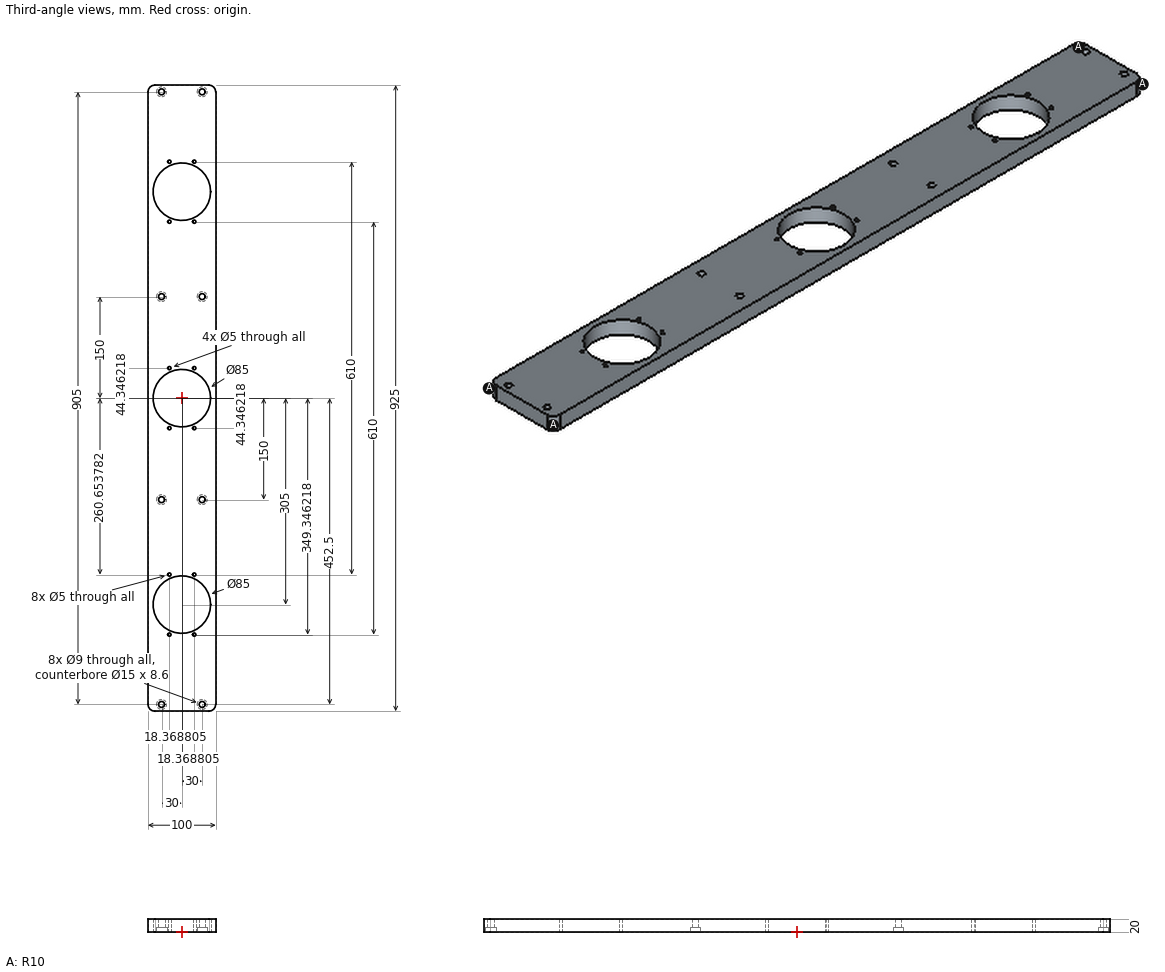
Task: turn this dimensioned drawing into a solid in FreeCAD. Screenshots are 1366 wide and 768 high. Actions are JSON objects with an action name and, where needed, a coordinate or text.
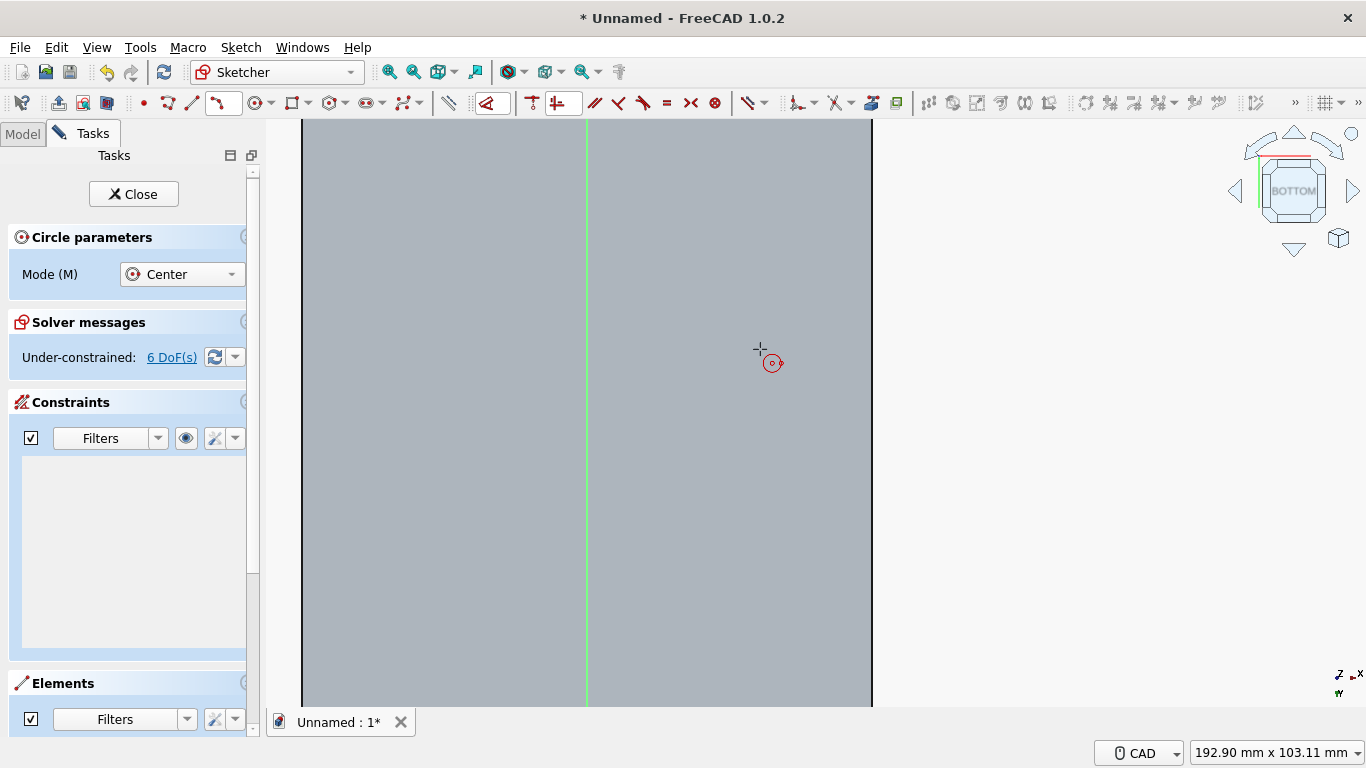
{"action": "scroll", "coordinate": [760, 349], "scroll_direction": "down", "scroll_amount": 13}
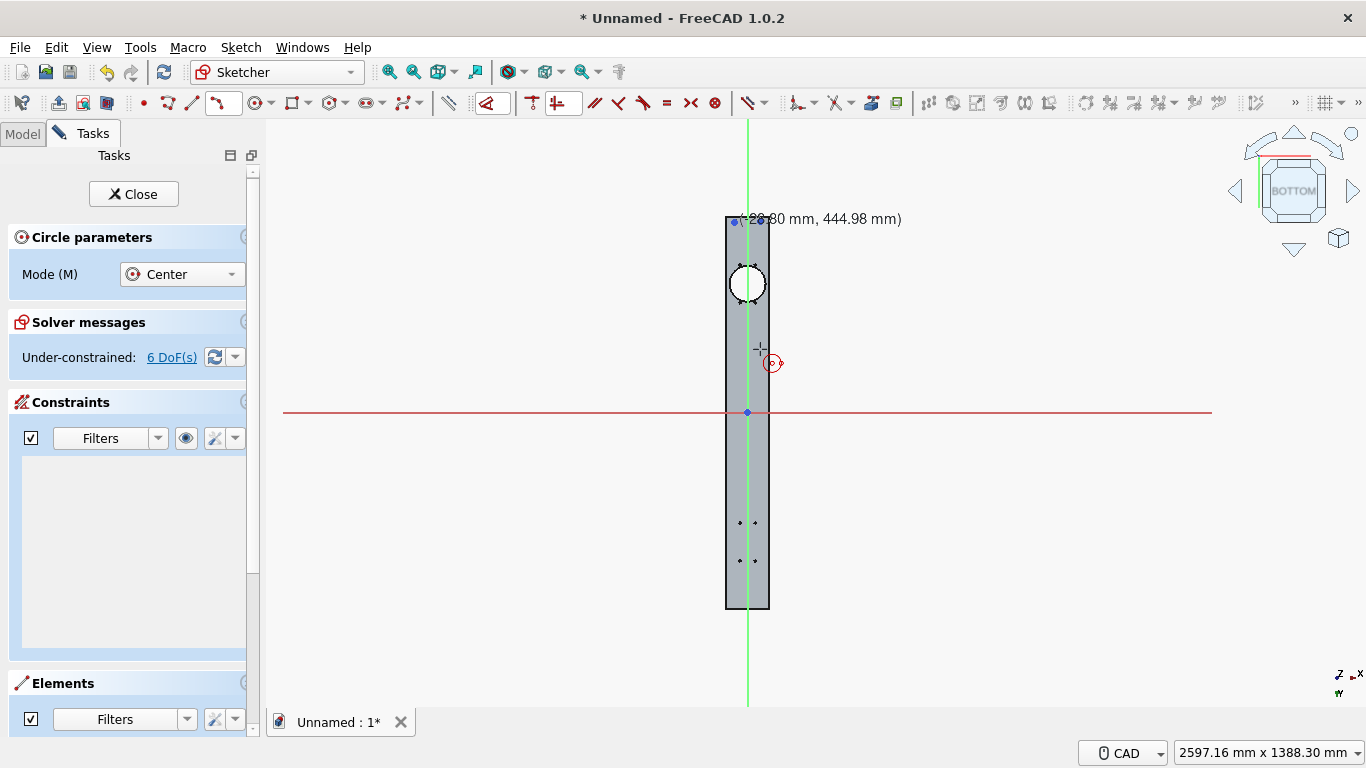
{"action": "scroll", "coordinate": [760, 349], "scroll_direction": "up", "scroll_amount": 2}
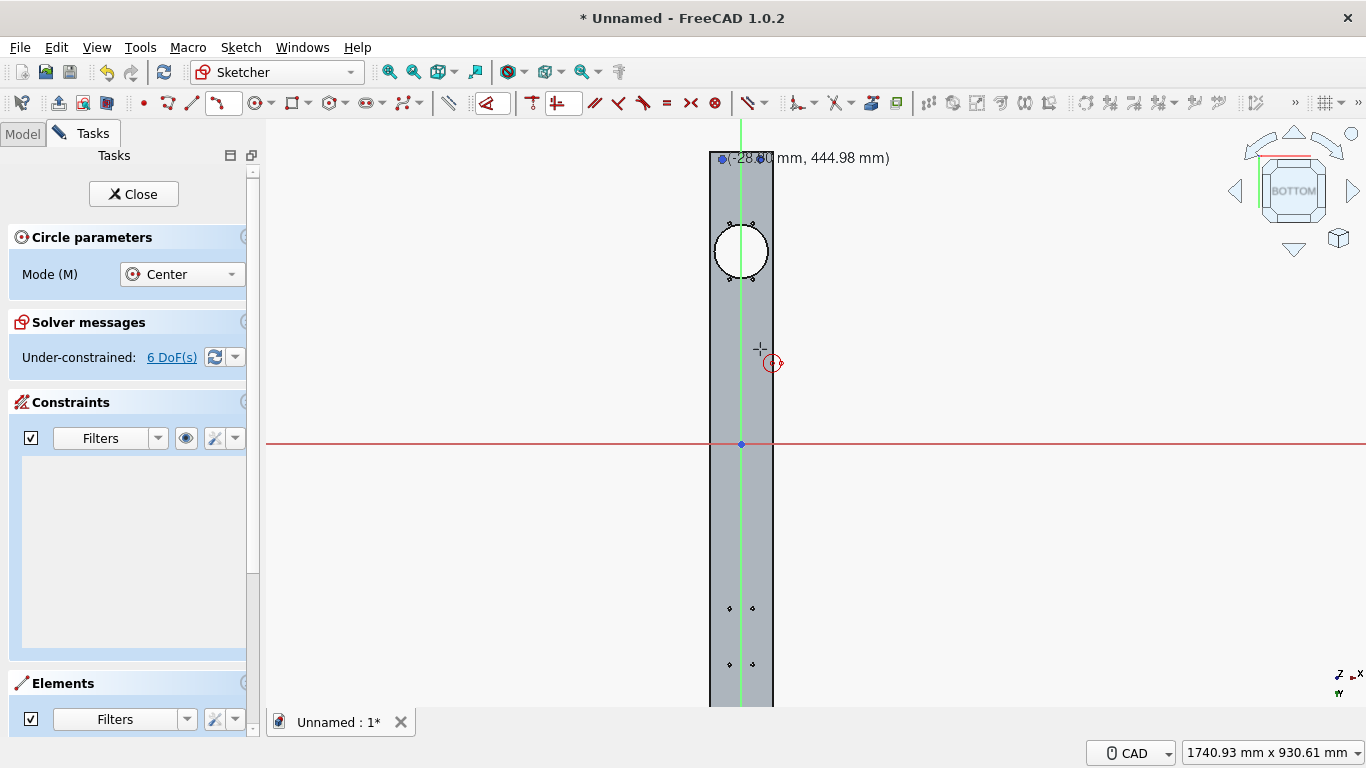
{"action": "left_click", "coordinate": [760, 349]}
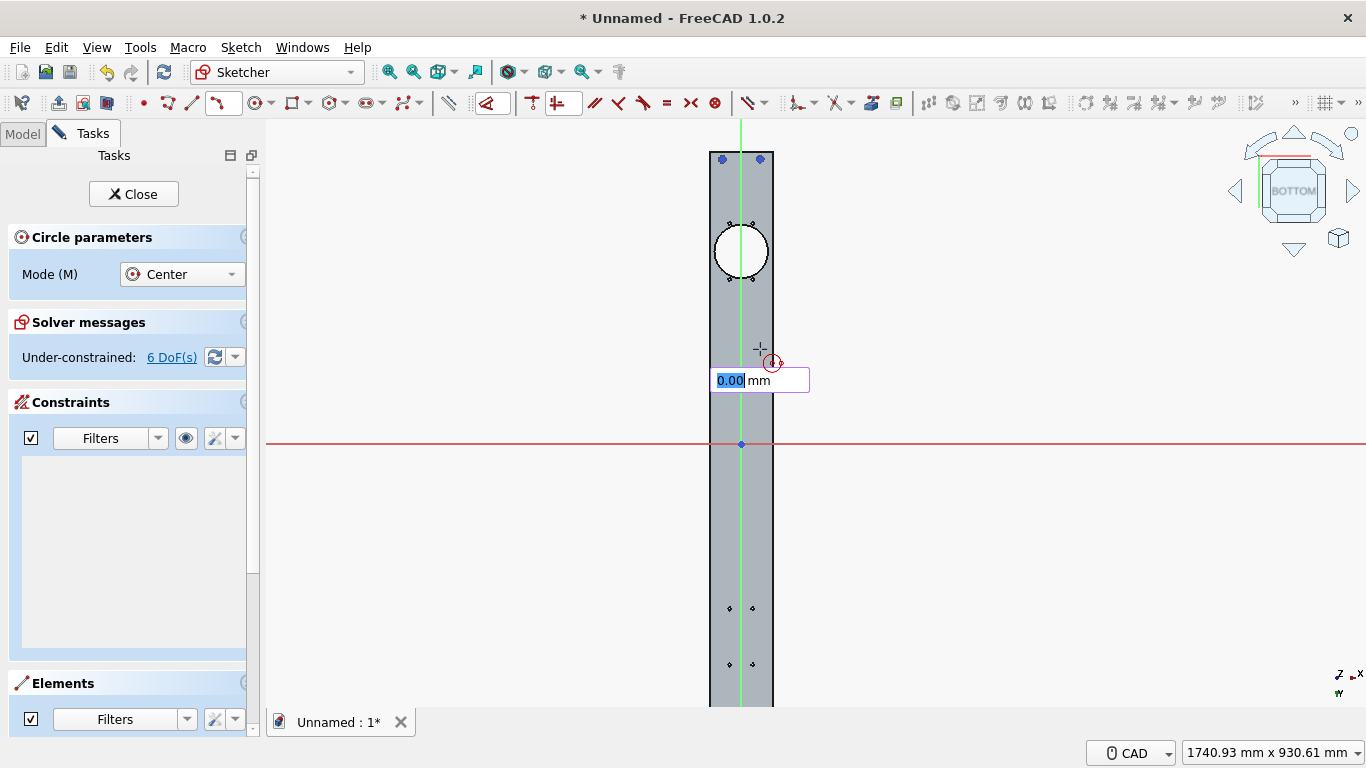
{"action": "scroll", "coordinate": [762, 347], "scroll_direction": "up", "scroll_amount": 9}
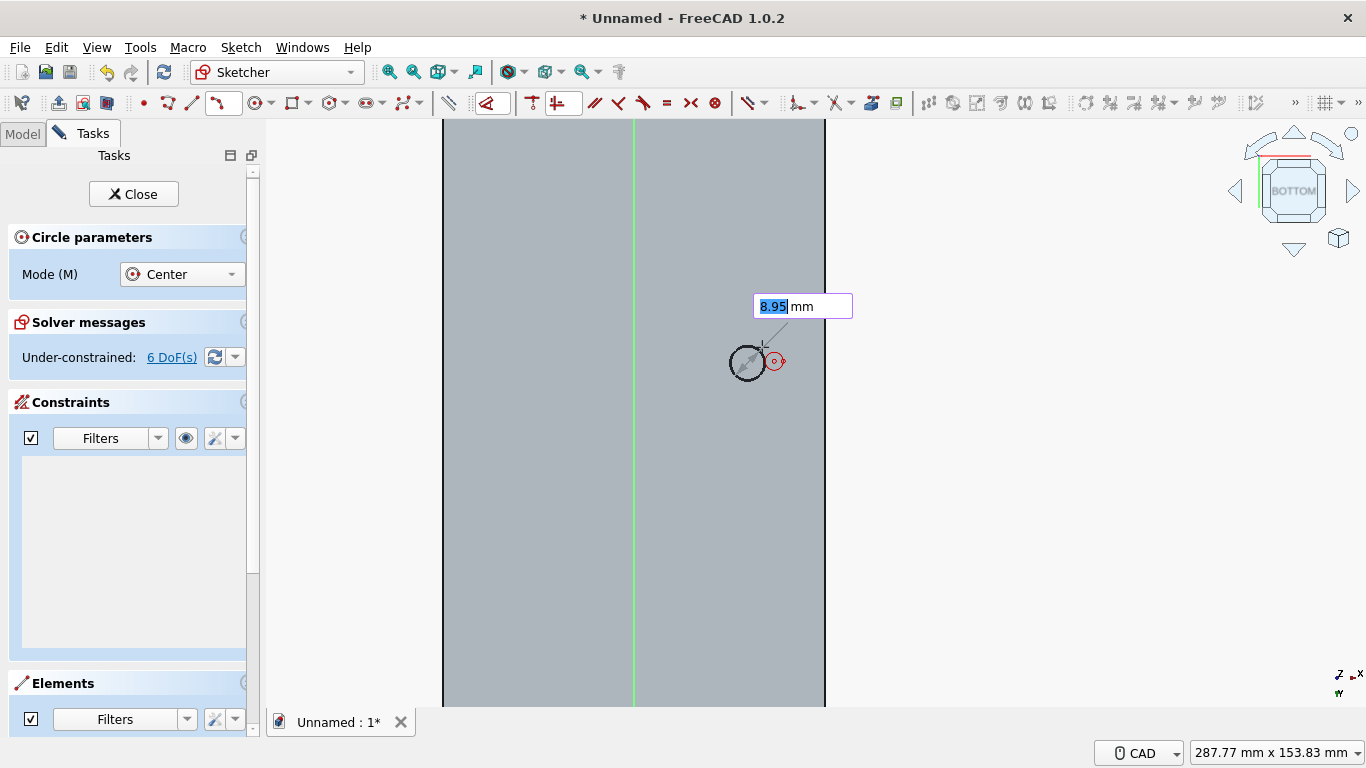
{"action": "left_click", "coordinate": [761, 347]}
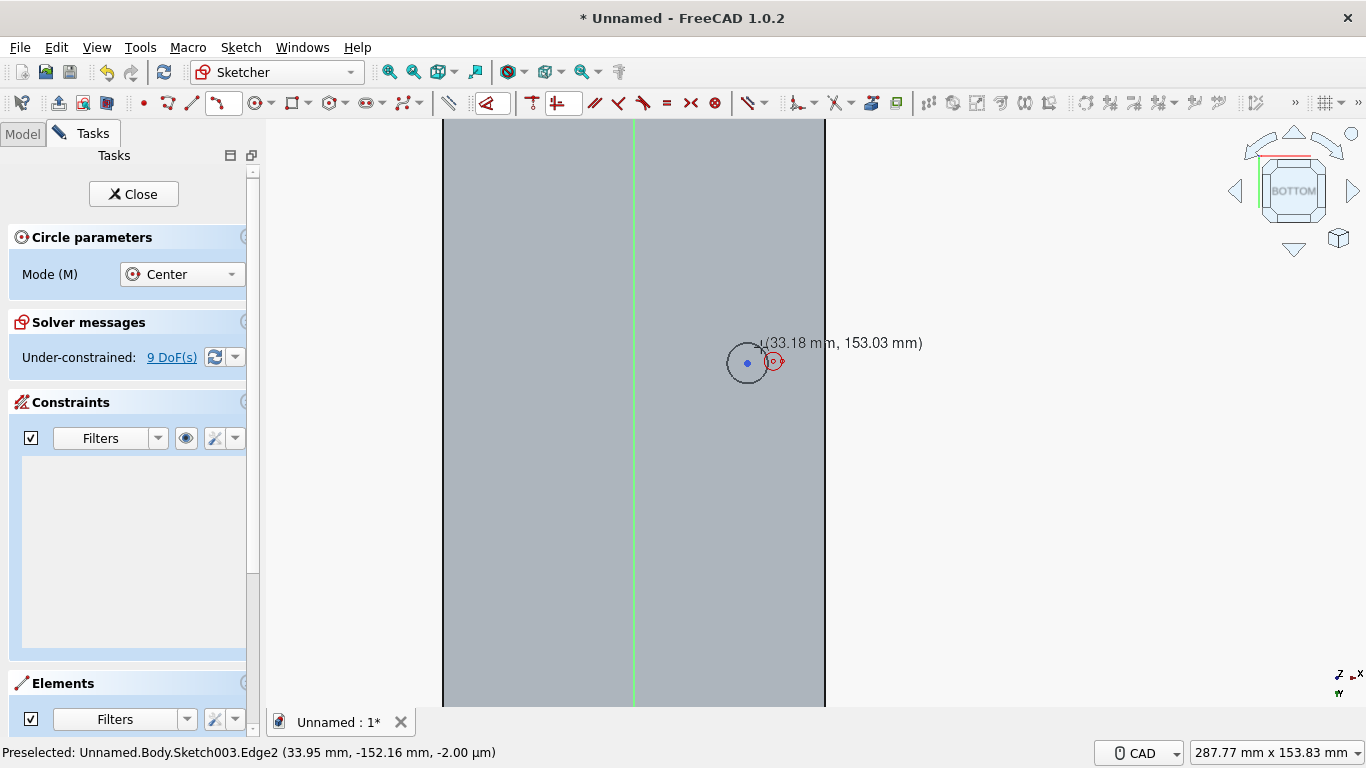
{"action": "scroll", "coordinate": [520, 360], "scroll_direction": "up", "scroll_amount": 2}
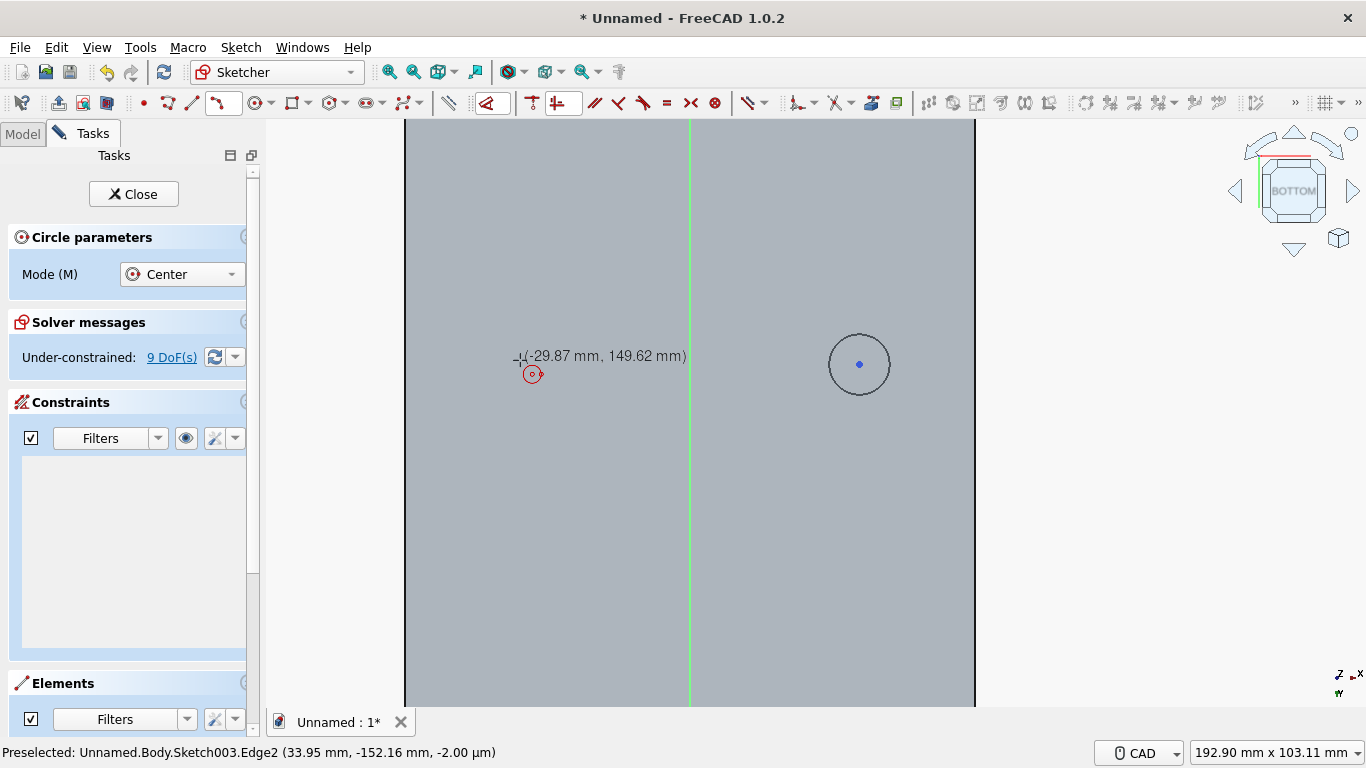
{"action": "scroll", "coordinate": [752, 349], "scroll_direction": "down", "scroll_amount": 13}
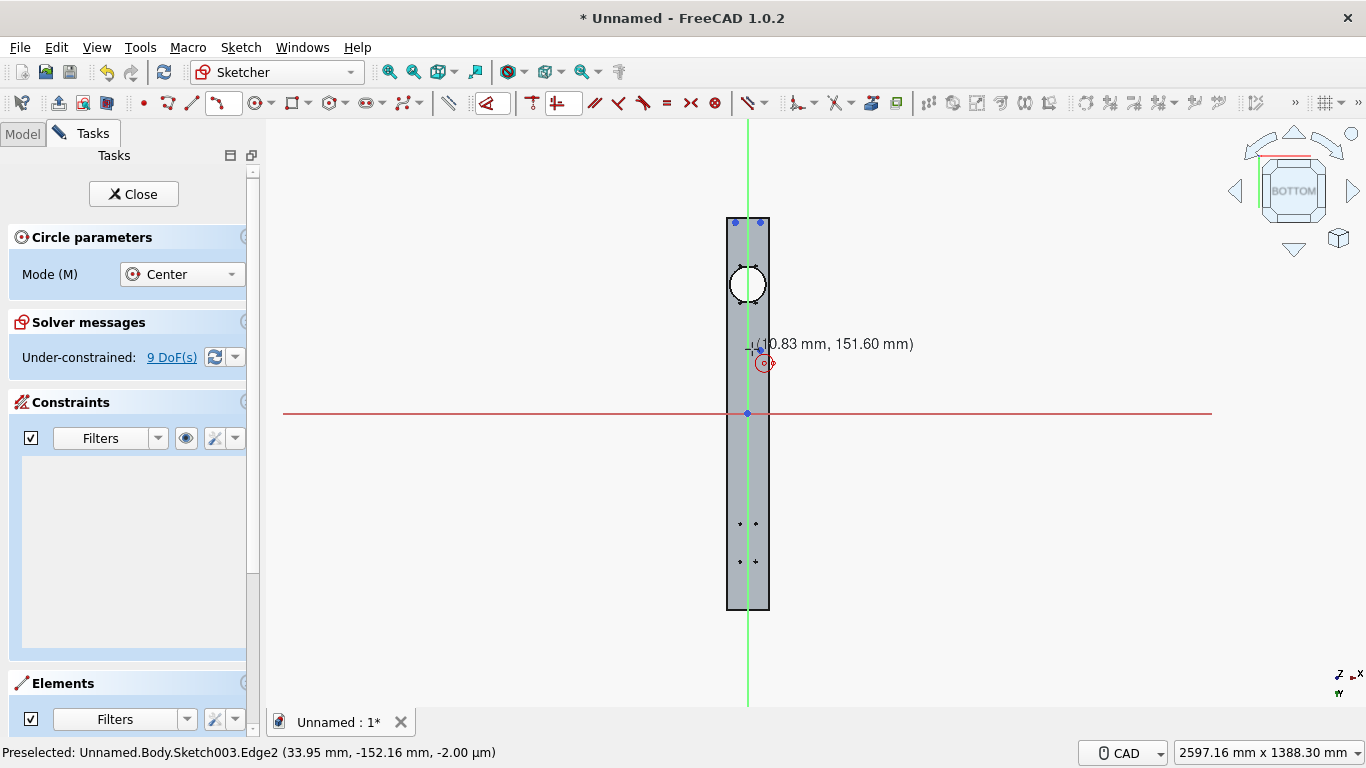
{"action": "scroll", "coordinate": [735, 350], "scroll_direction": "up", "scroll_amount": 2}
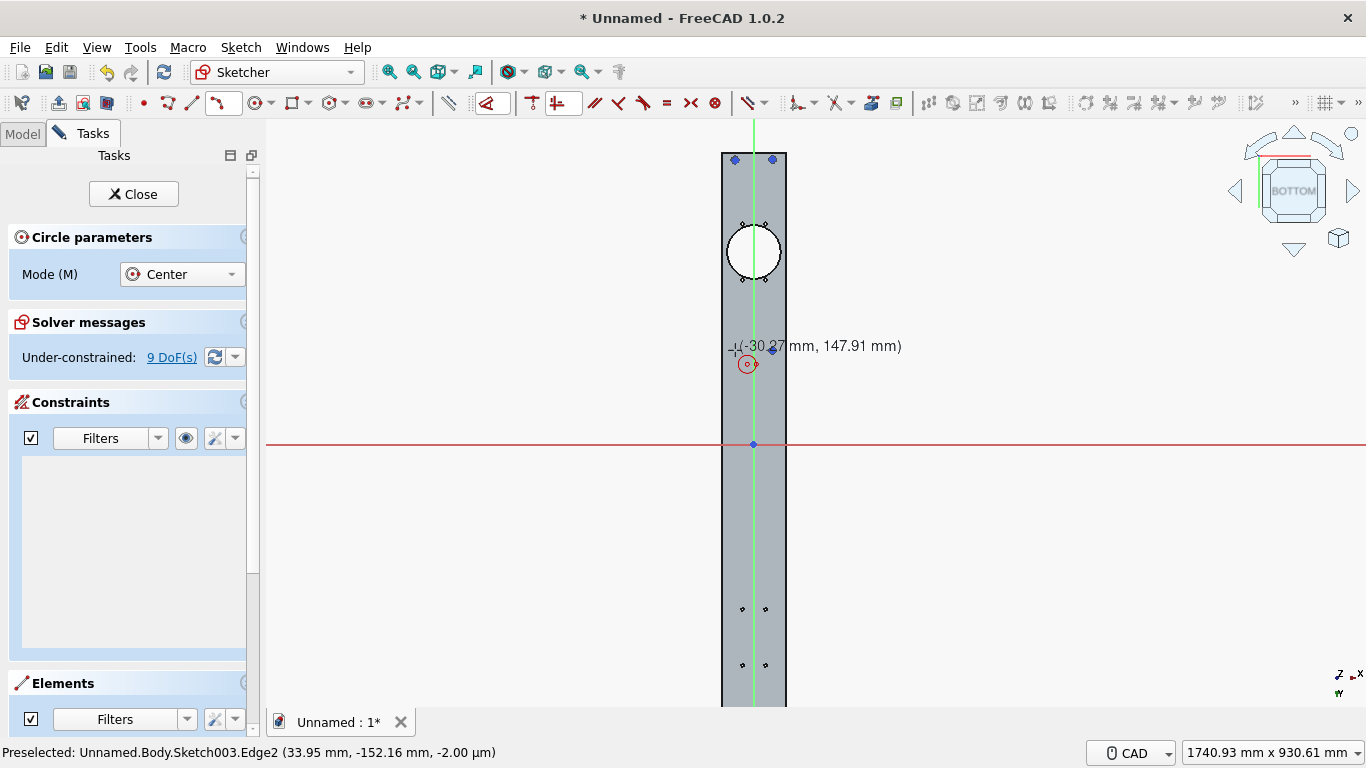
{"action": "left_click", "coordinate": [735, 350]}